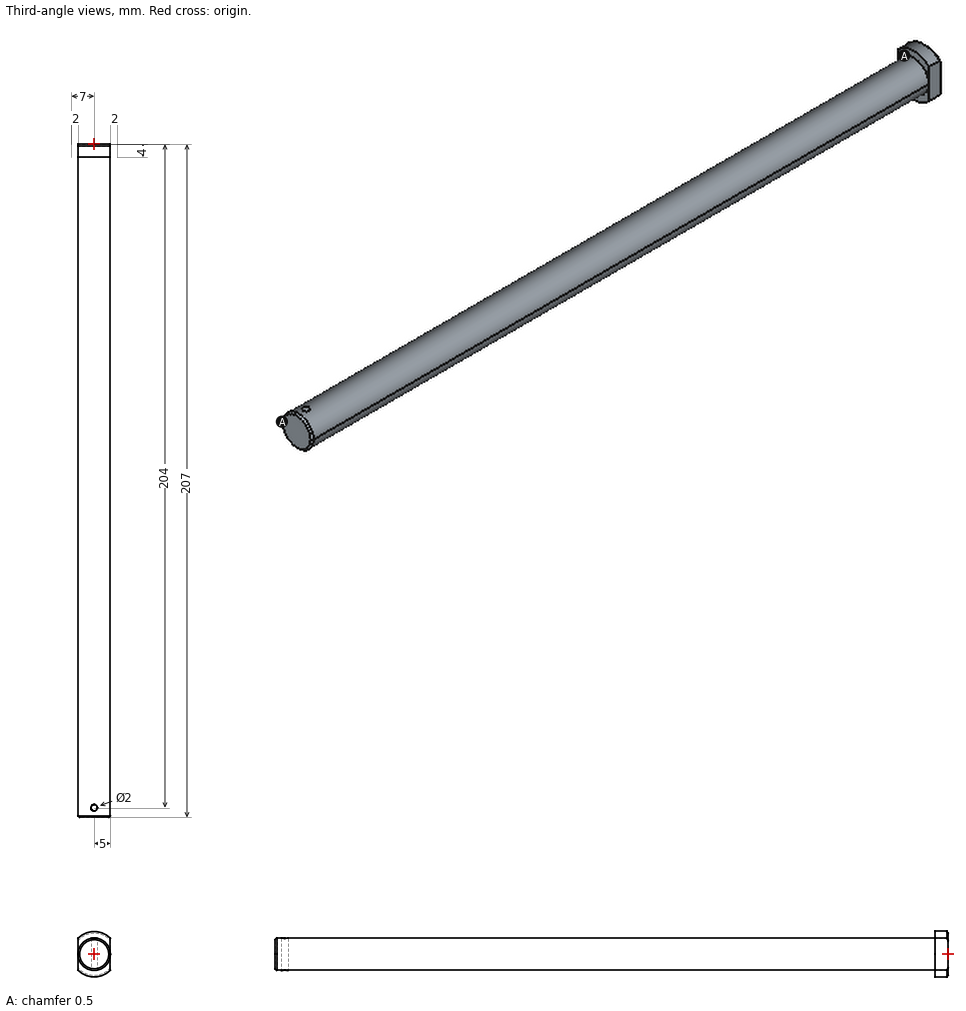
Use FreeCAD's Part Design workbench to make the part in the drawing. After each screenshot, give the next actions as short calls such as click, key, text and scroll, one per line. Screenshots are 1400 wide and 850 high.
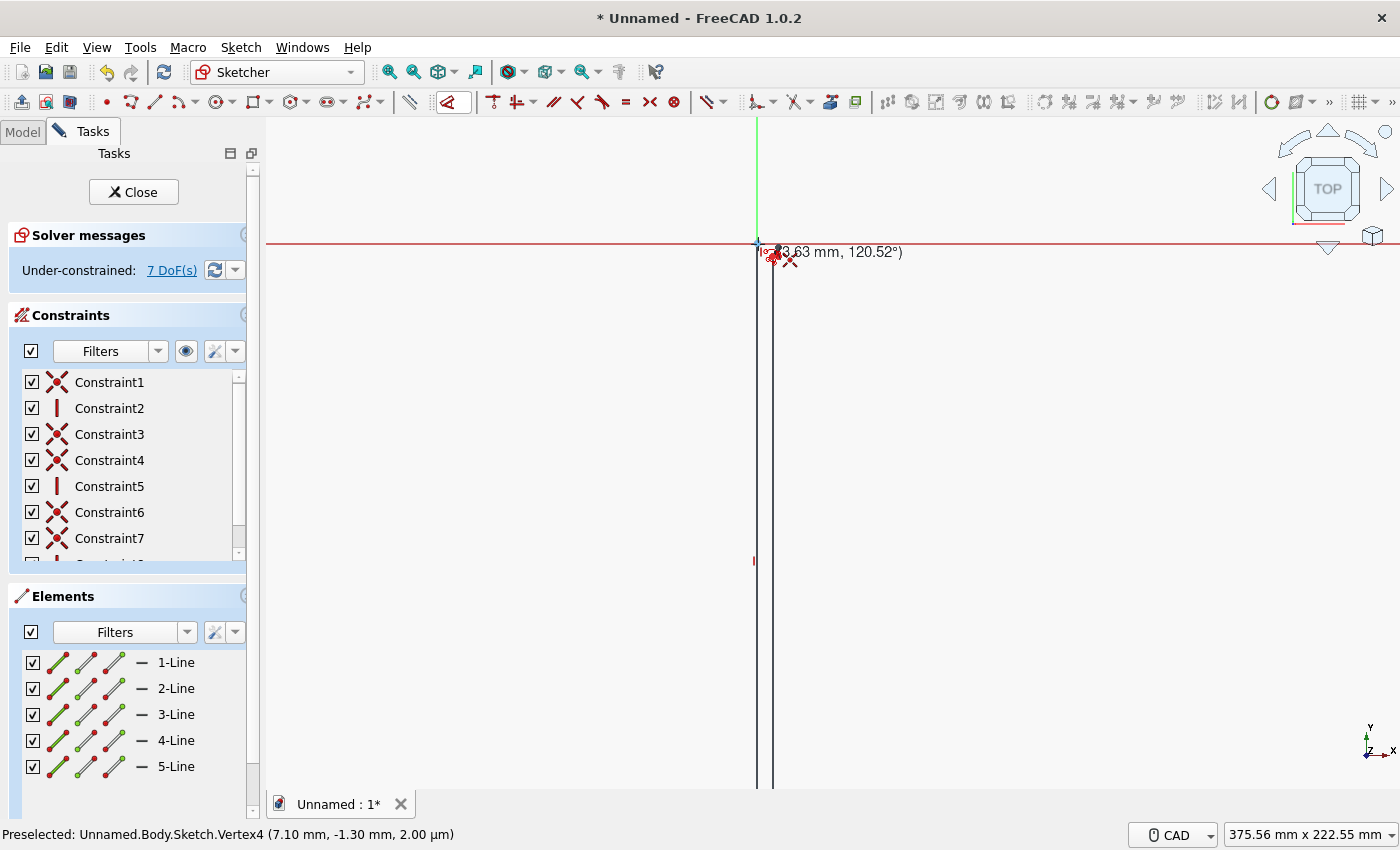
click(757, 244)
key(Escape)
key(Escape)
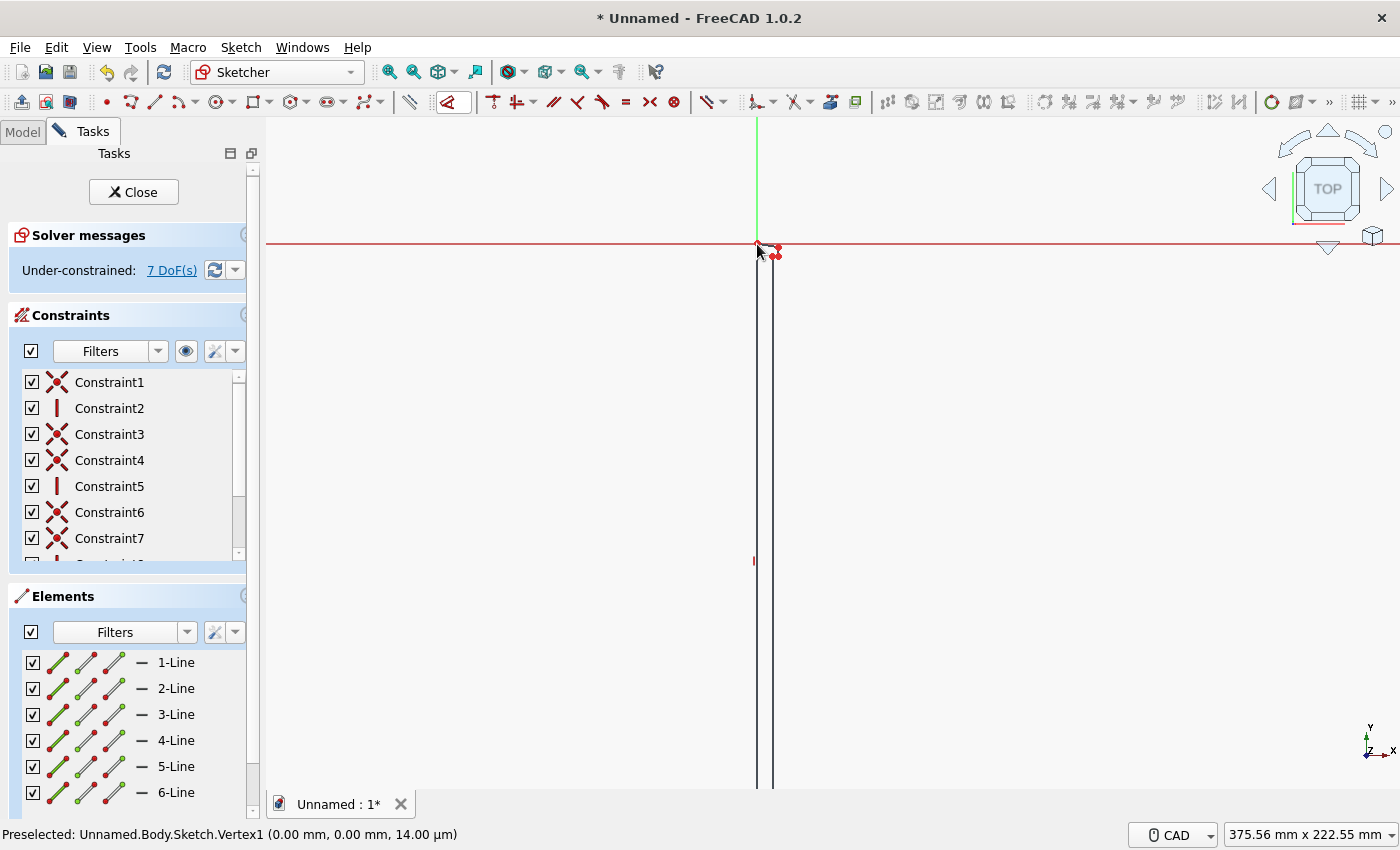
scroll(758, 243, down, 2)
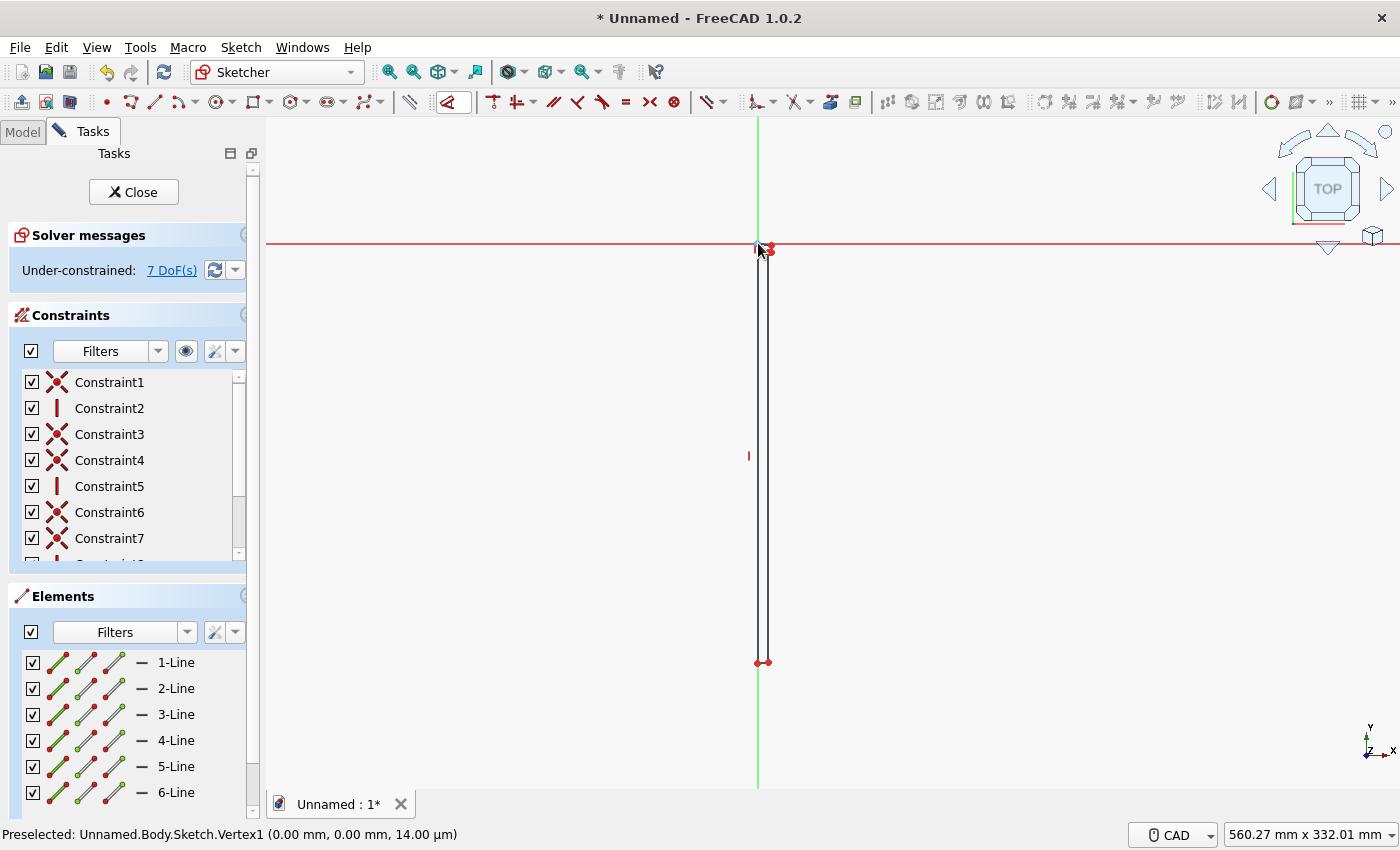
scroll(763, 663, up, 5)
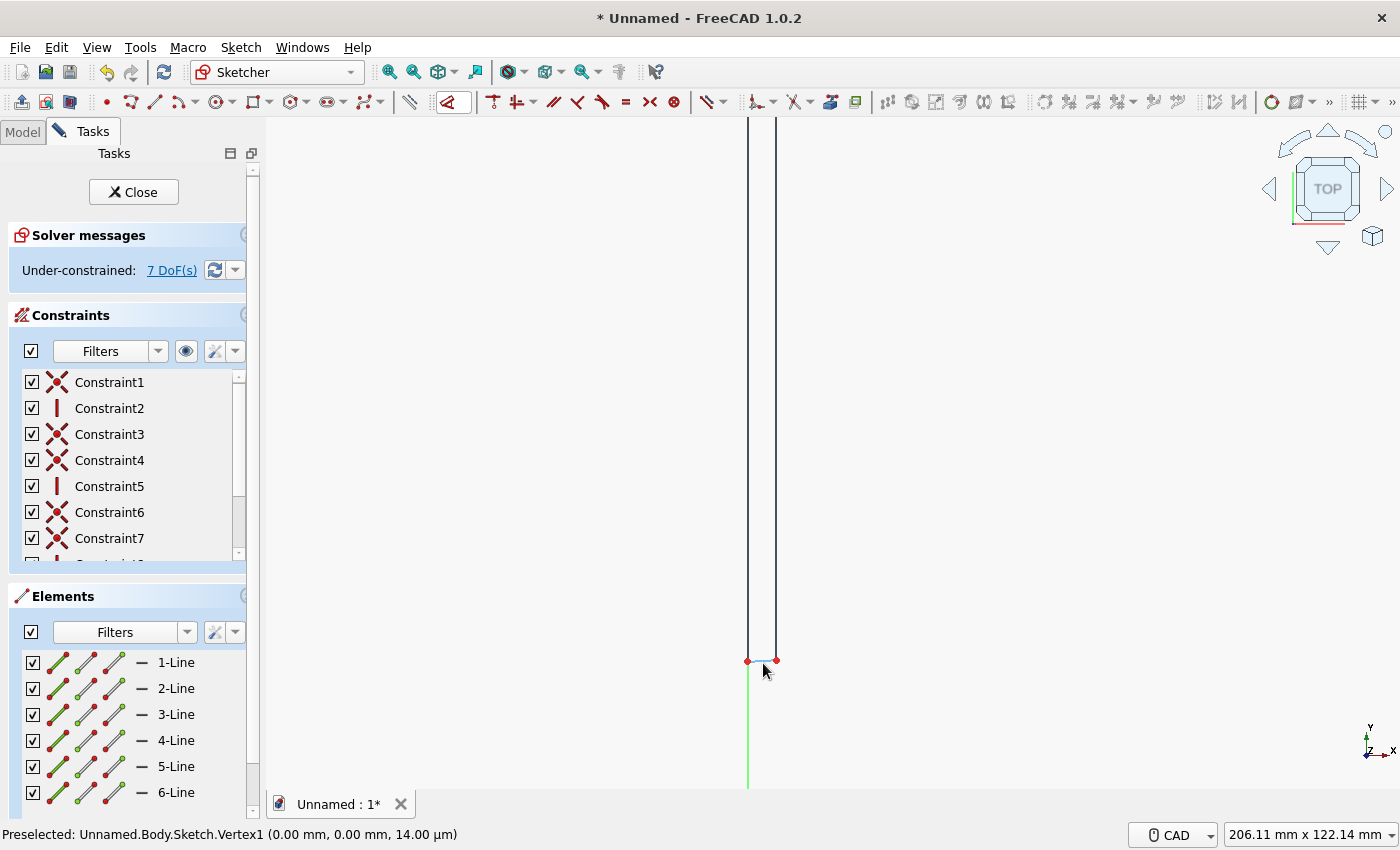
click(762, 661)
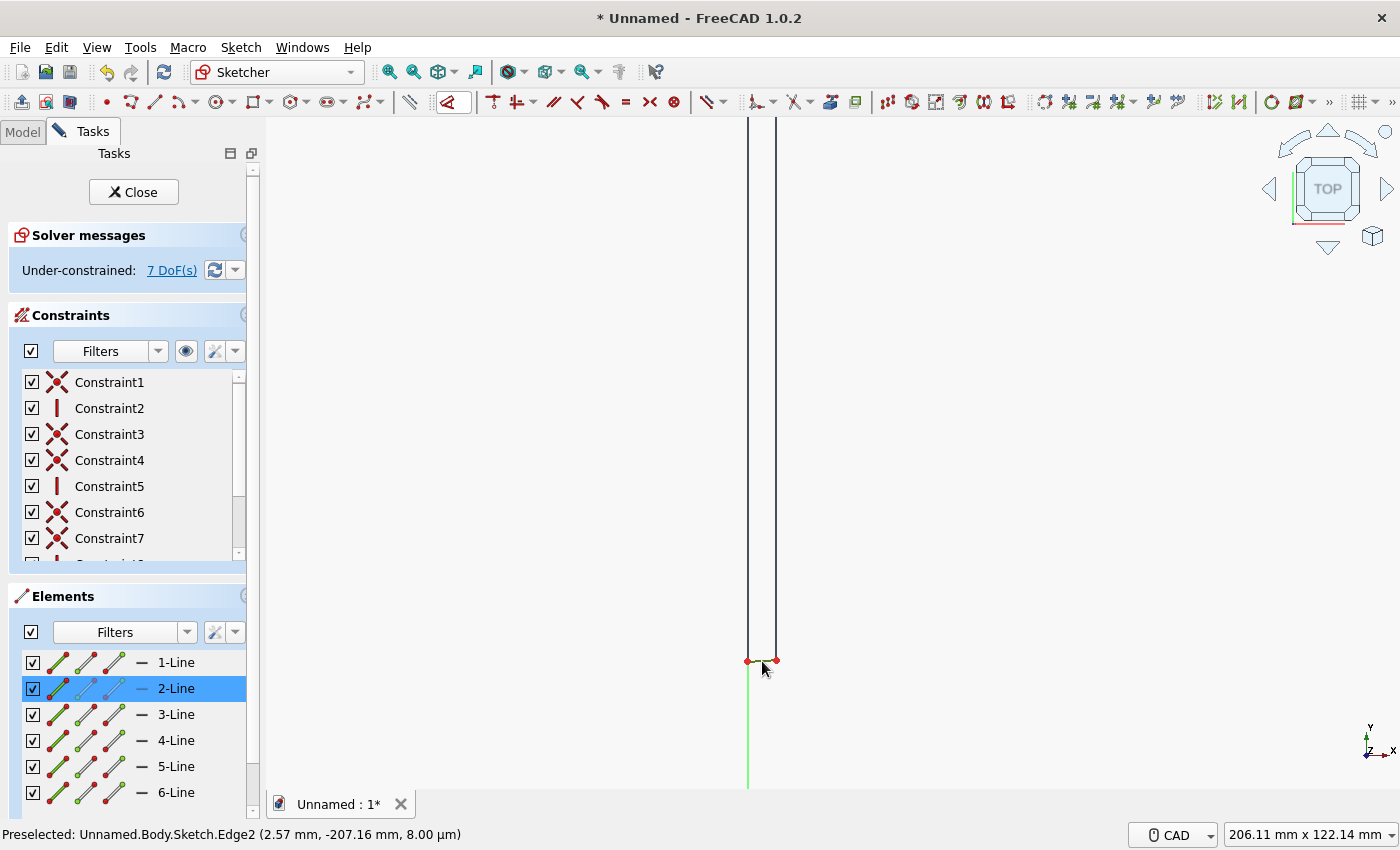
click(536, 102)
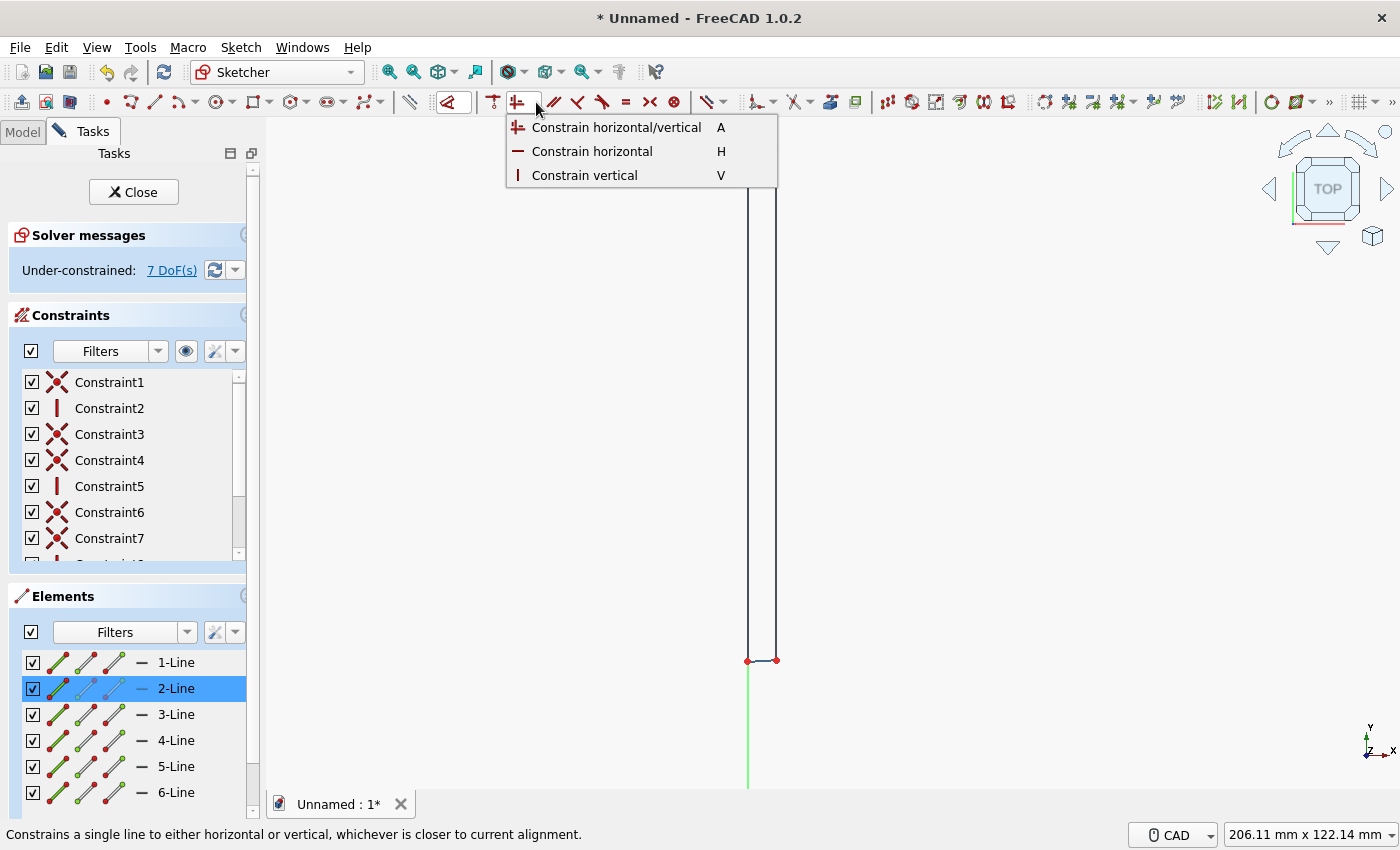
click(642, 151)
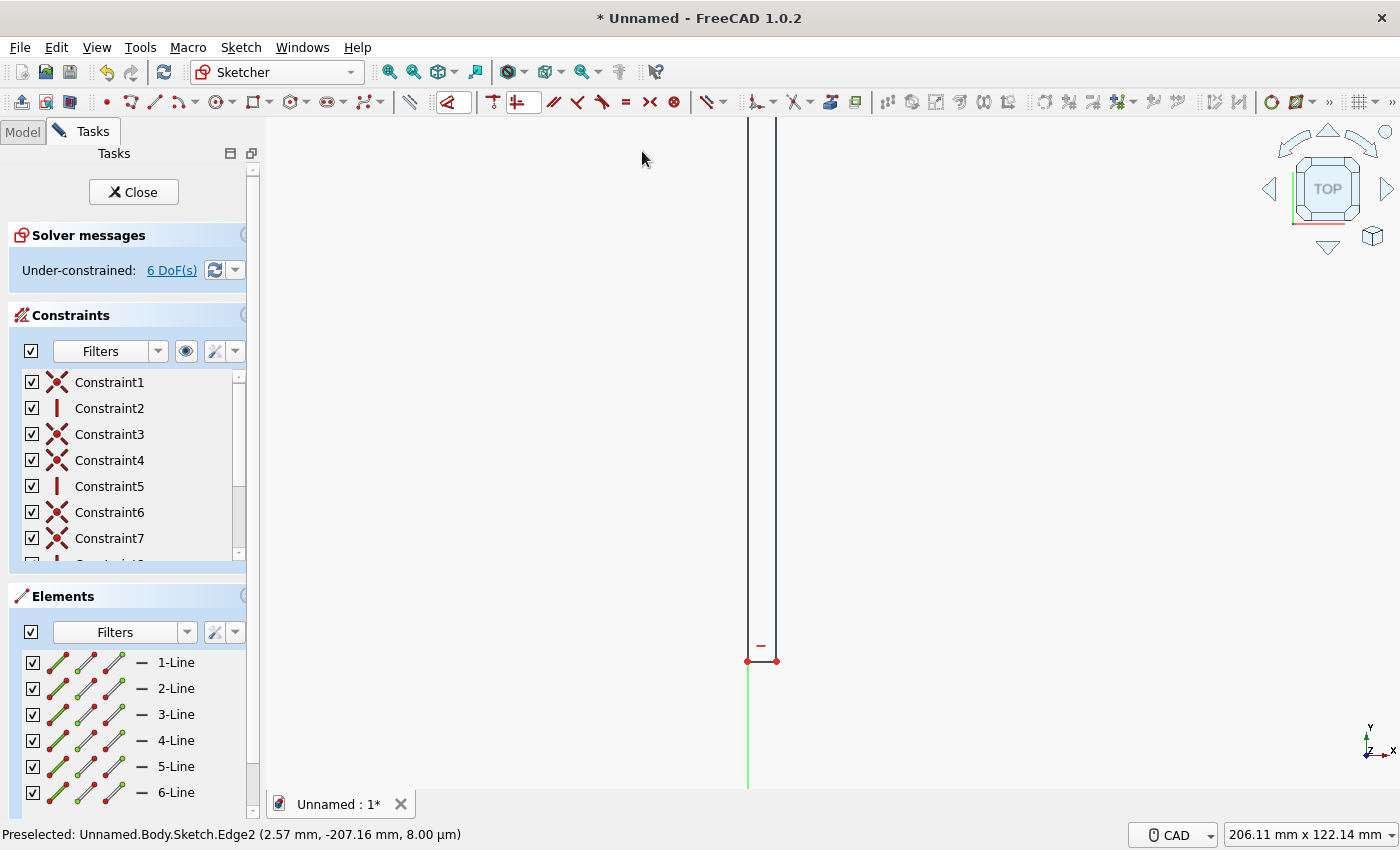
scroll(763, 664, down, 5)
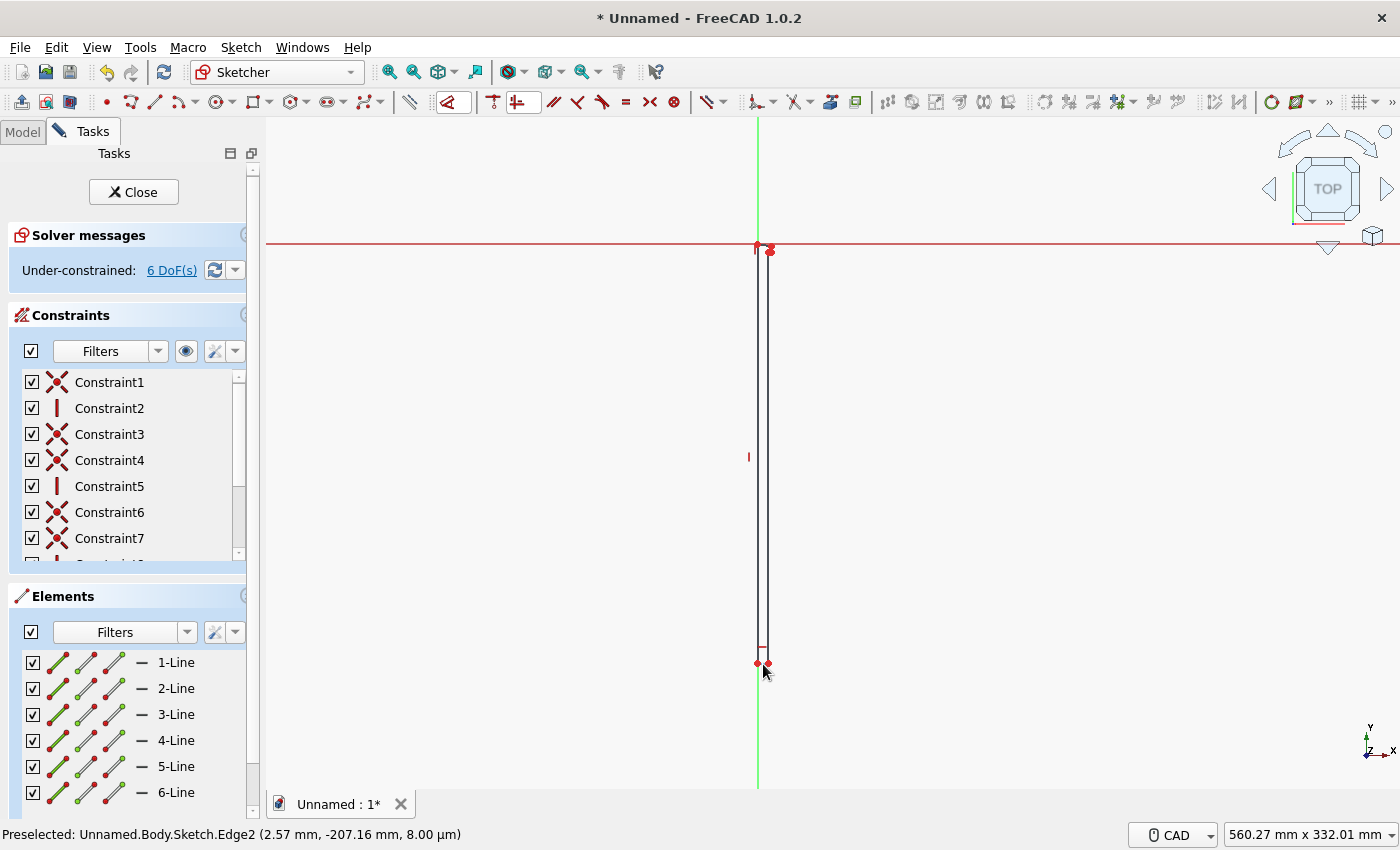
scroll(770, 253, up, 11)